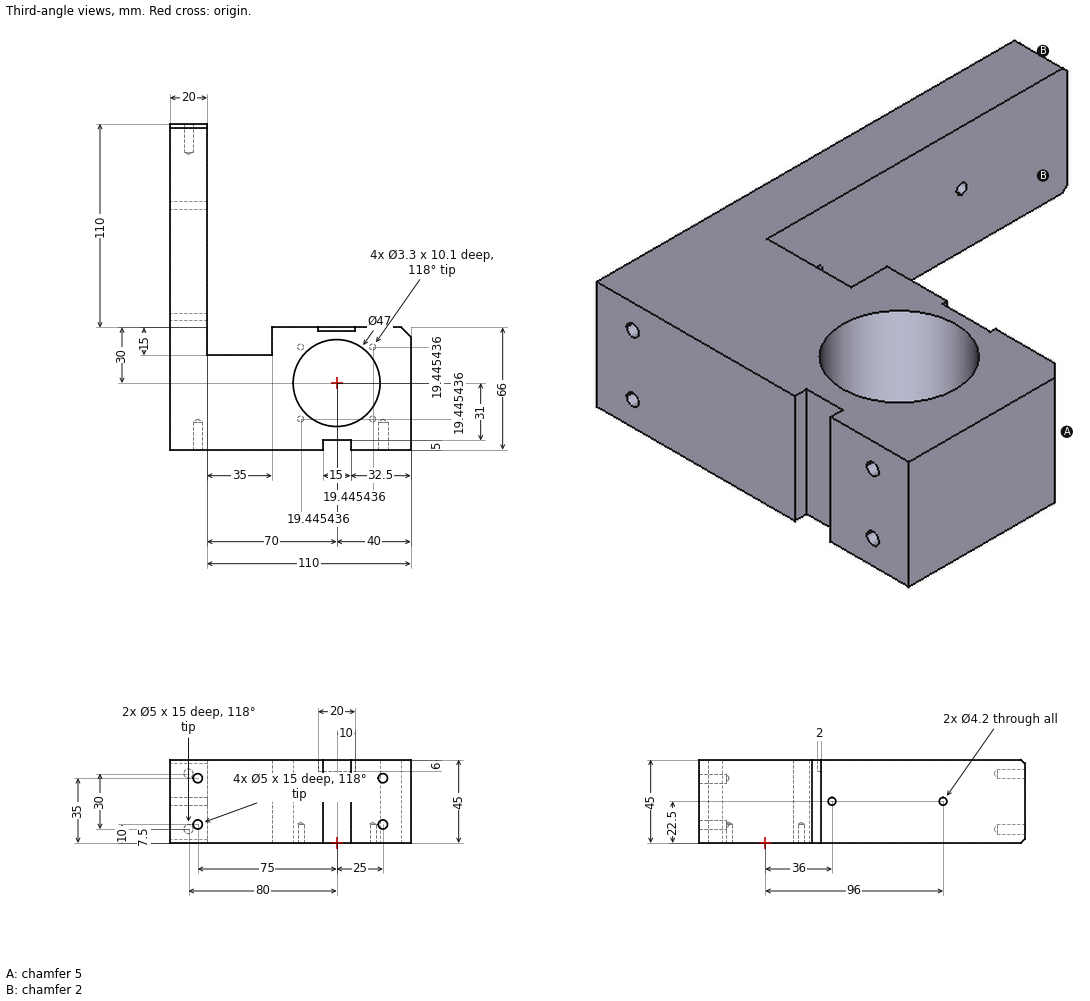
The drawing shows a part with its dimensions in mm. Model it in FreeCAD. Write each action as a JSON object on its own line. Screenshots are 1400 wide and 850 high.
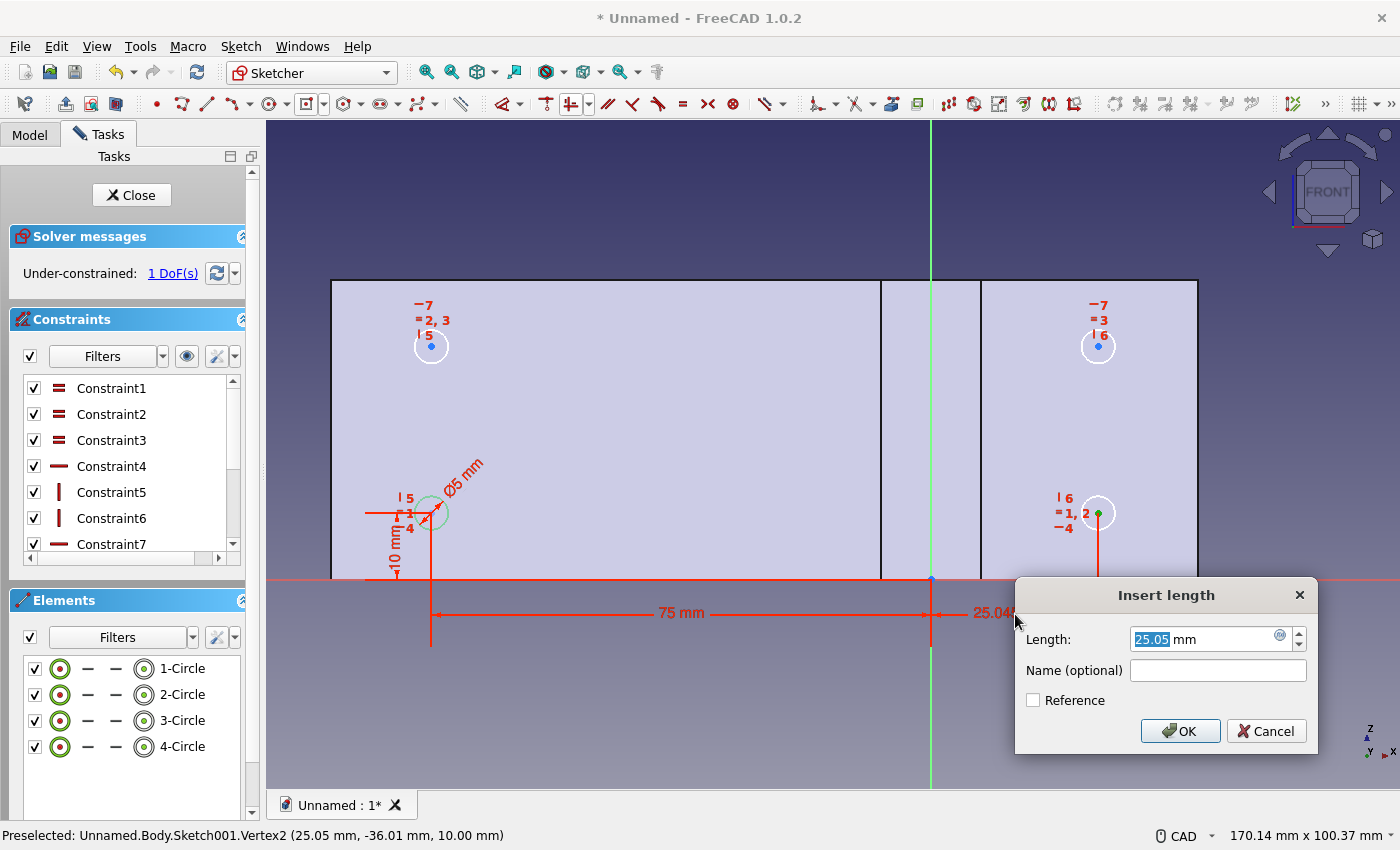
{"action": "type", "text": "25"}
{"action": "key", "text": "Return"}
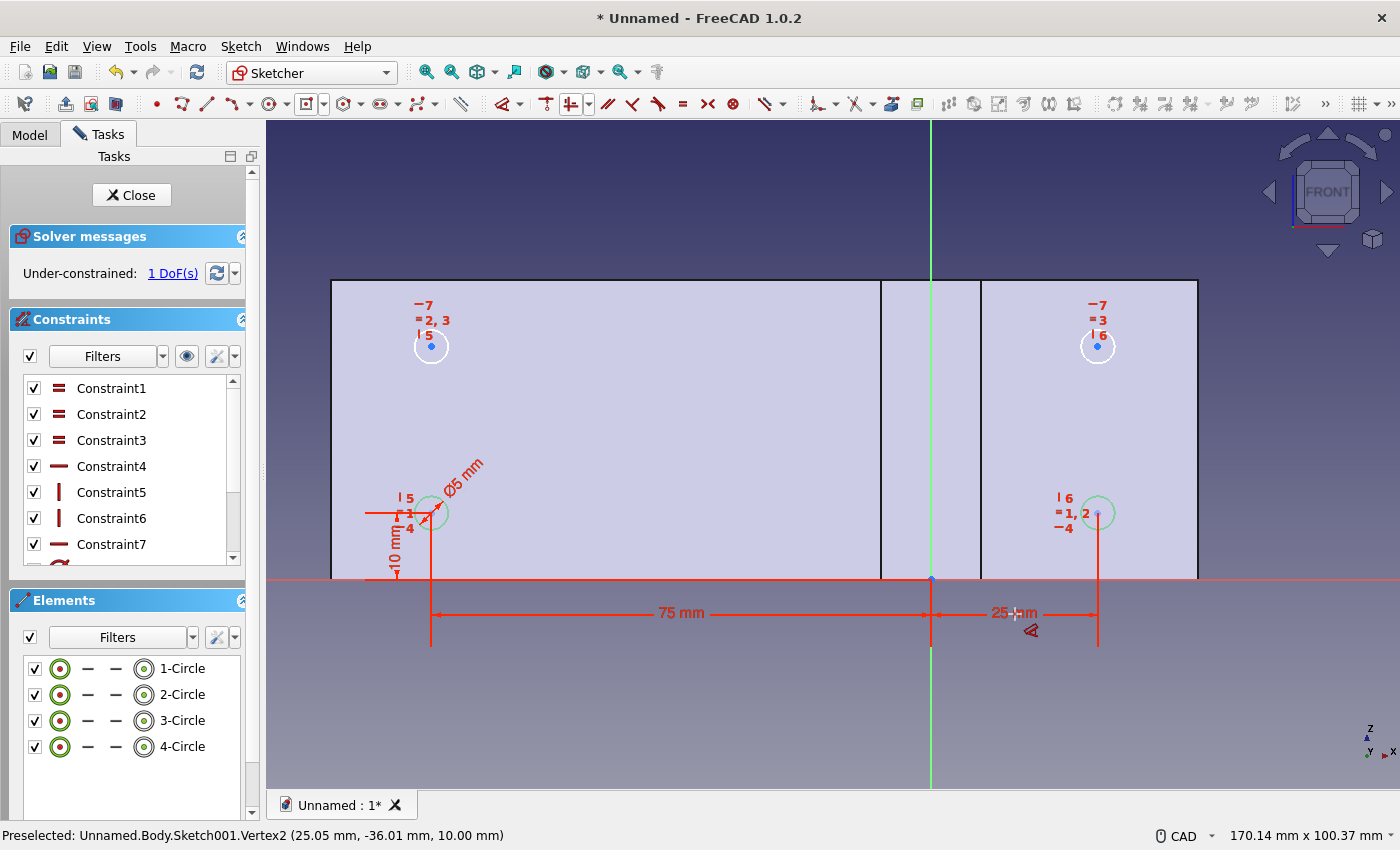
{"action": "left_click", "coordinate": [431, 347]}
{"action": "left_click", "coordinate": [397, 410]}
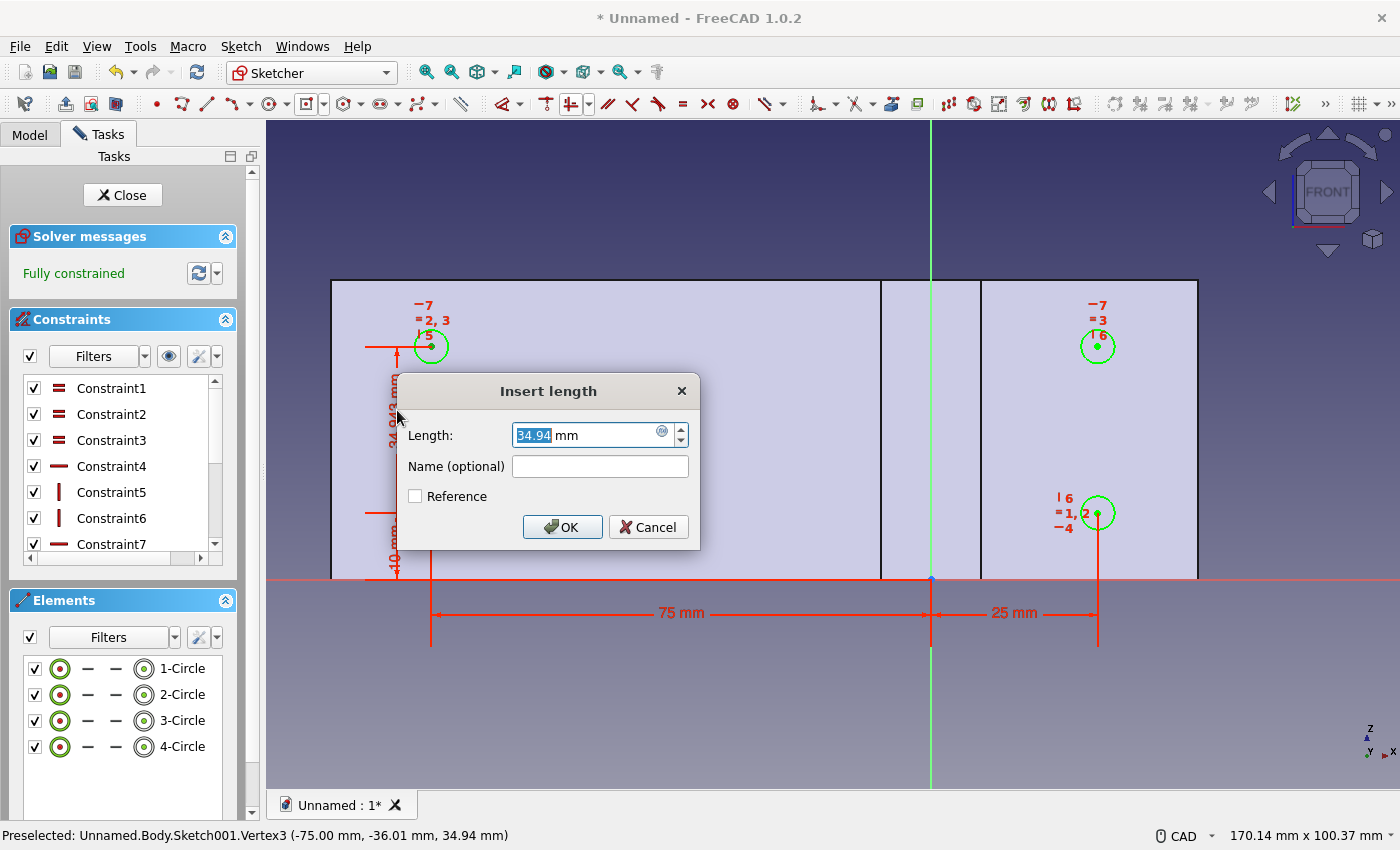
{"action": "type", "text": "35"}
{"action": "key", "text": "Return"}
{"action": "key", "text": "Escape"}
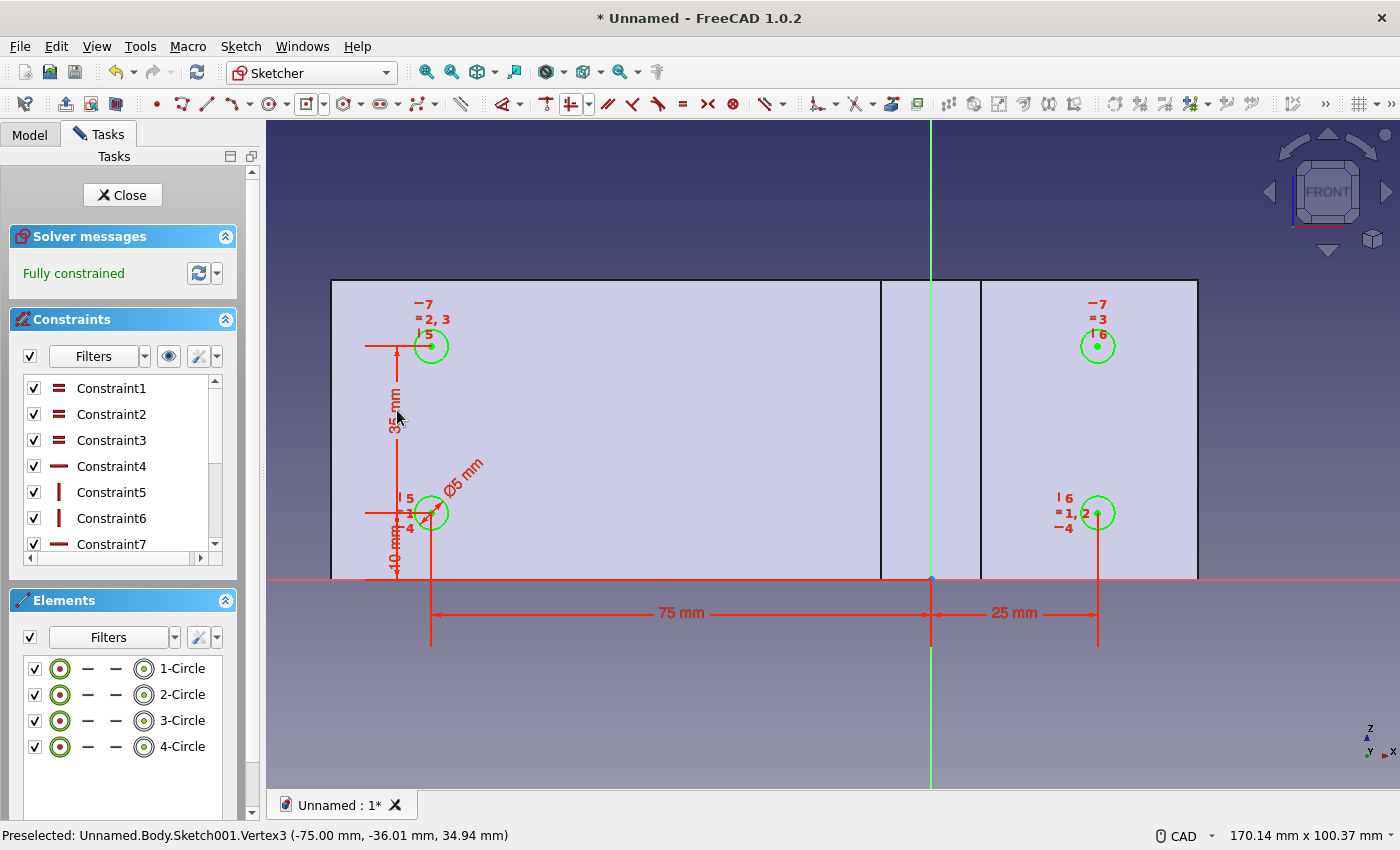
{"action": "left_click", "coordinate": [123, 195]}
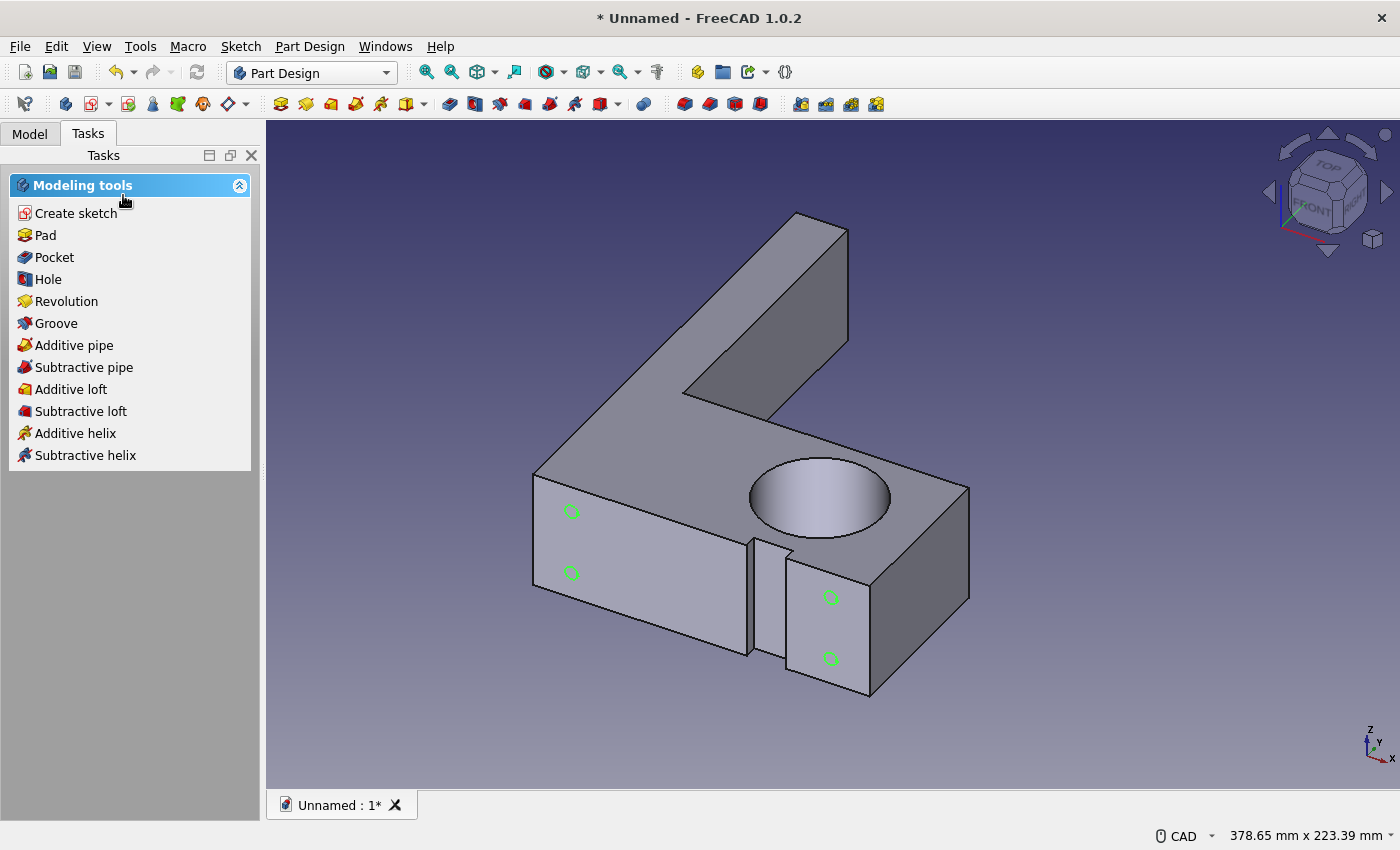
{"action": "left_click", "coordinate": [475, 104]}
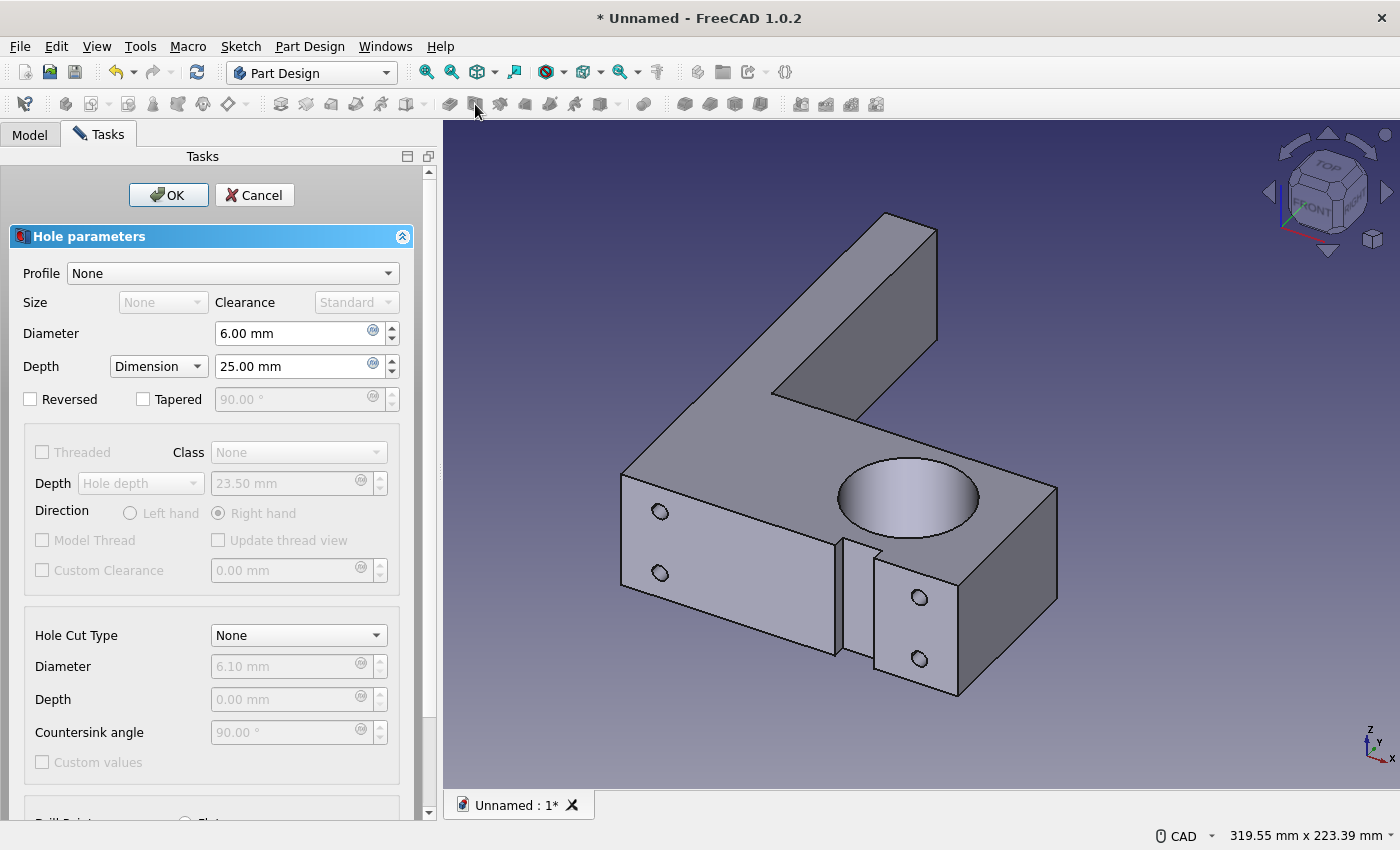
{"action": "triple_click", "coordinate": [300, 334]}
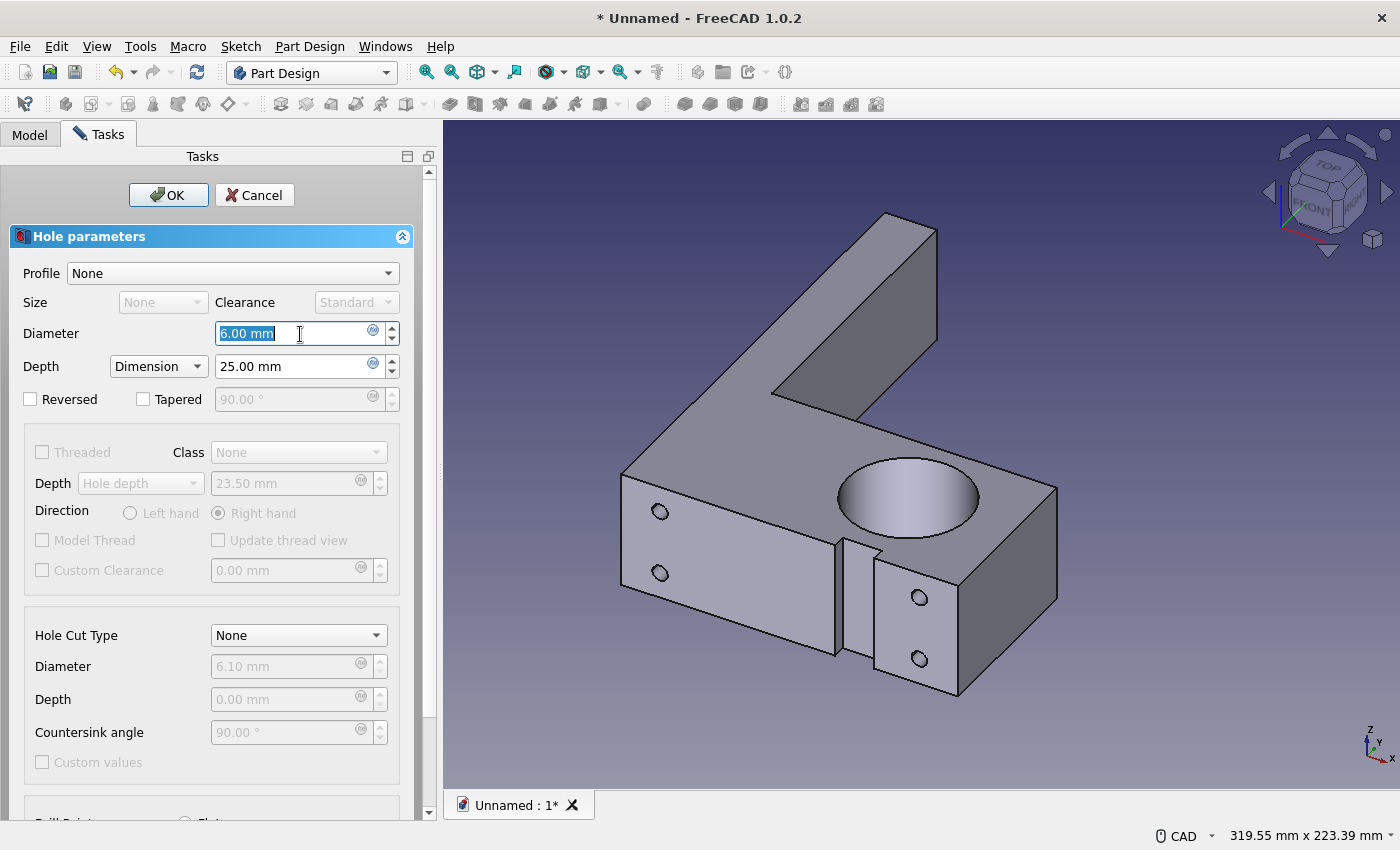
{"action": "type", "text": "5"}
{"action": "key", "text": "Tab"}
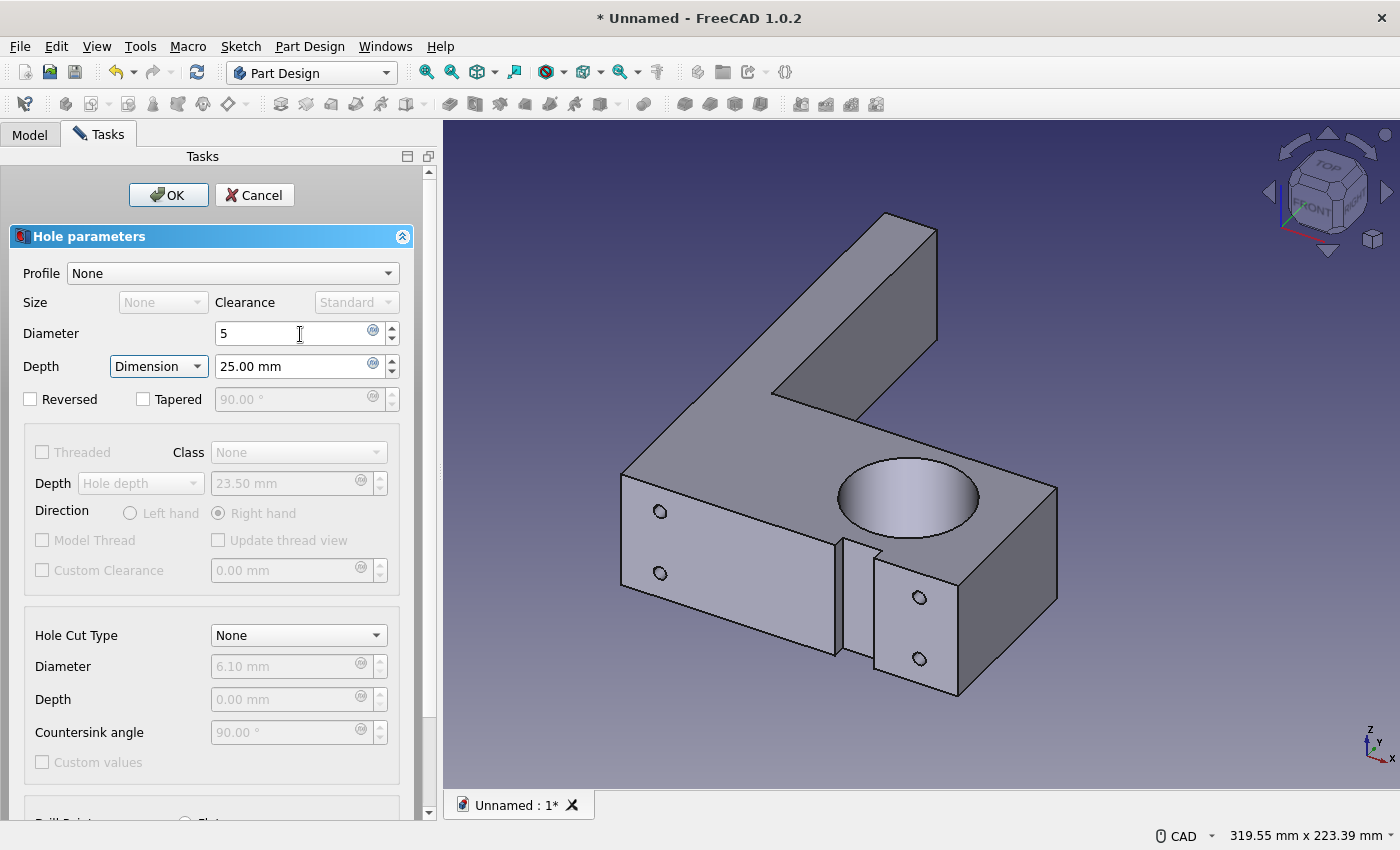
{"action": "triple_click", "coordinate": [300, 366]}